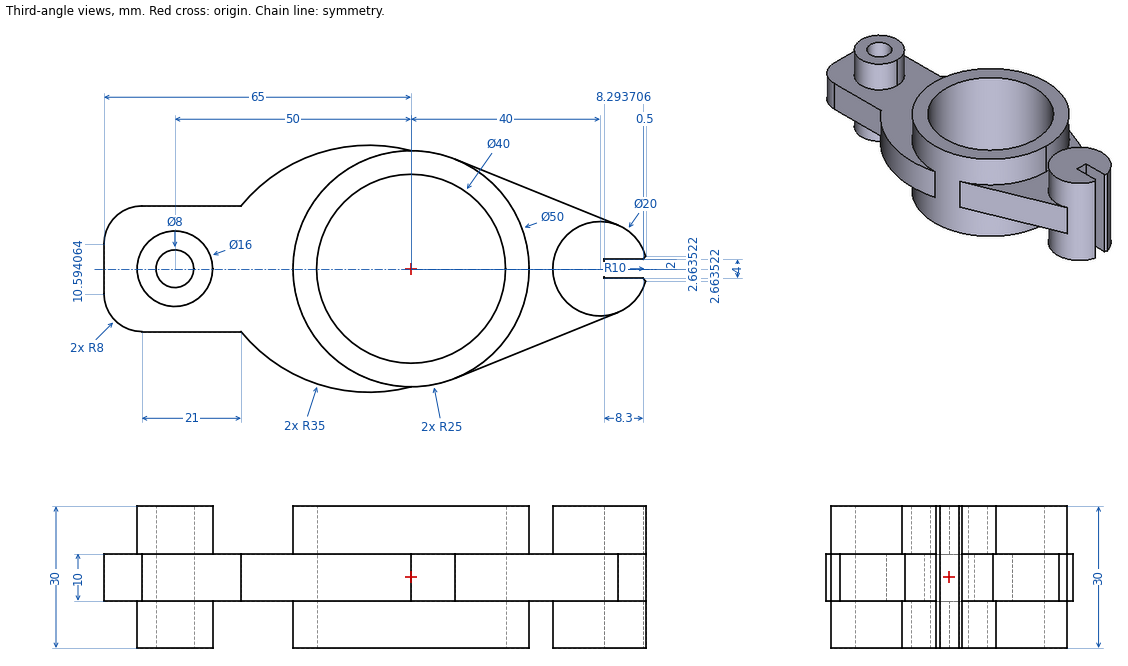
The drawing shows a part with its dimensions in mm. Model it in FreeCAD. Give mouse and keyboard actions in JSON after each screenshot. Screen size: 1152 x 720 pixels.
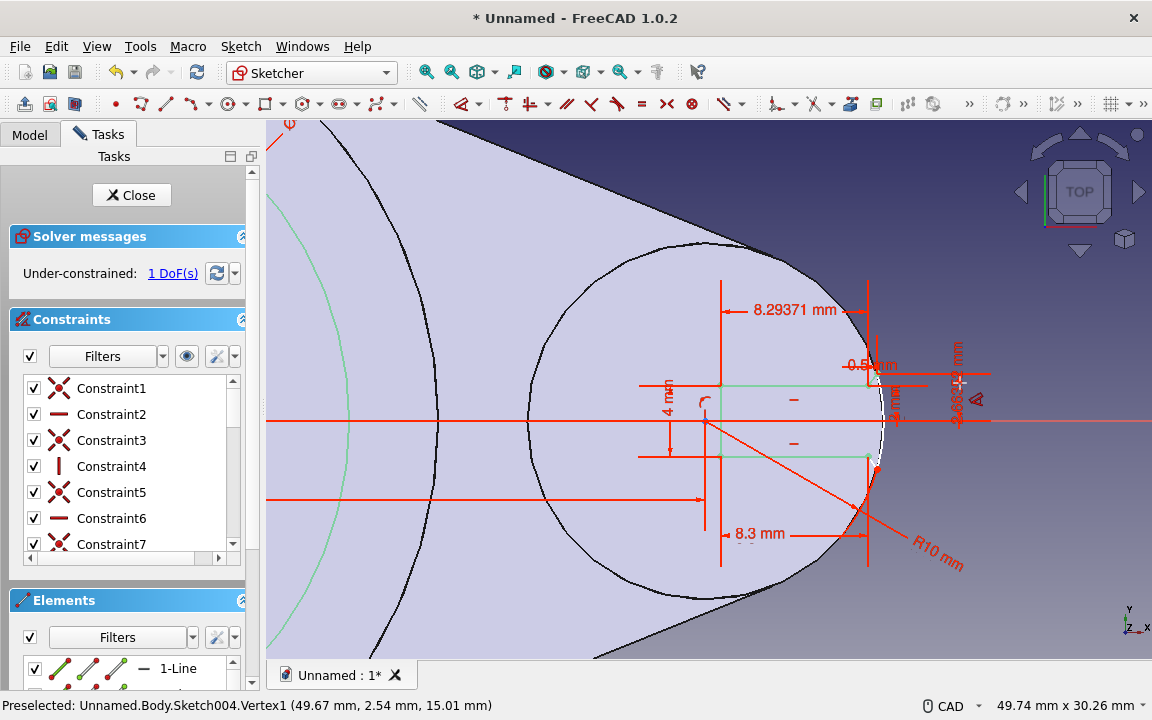
{"action": "left_click", "coordinate": [877, 469]}
{"action": "left_click", "coordinate": [911, 445]}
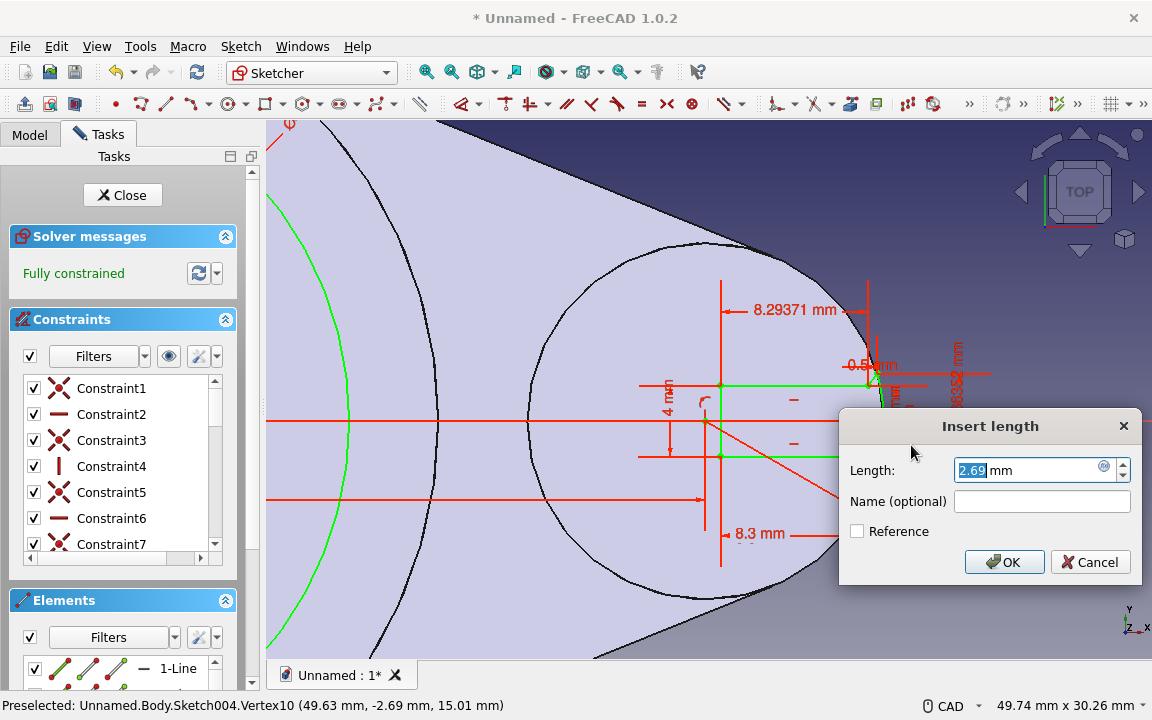
{"action": "type", "text": "2.663522"}
{"action": "key", "text": "Return"}
{"action": "key", "text": "Escape"}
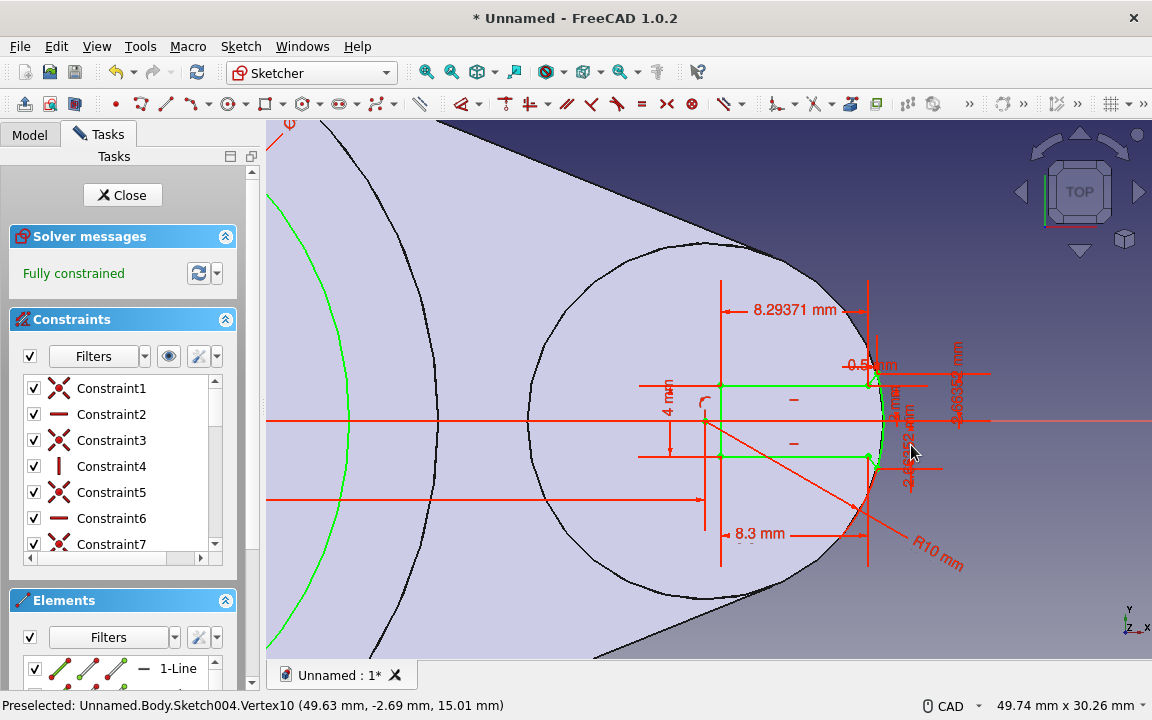
{"action": "left_click", "coordinate": [123, 195]}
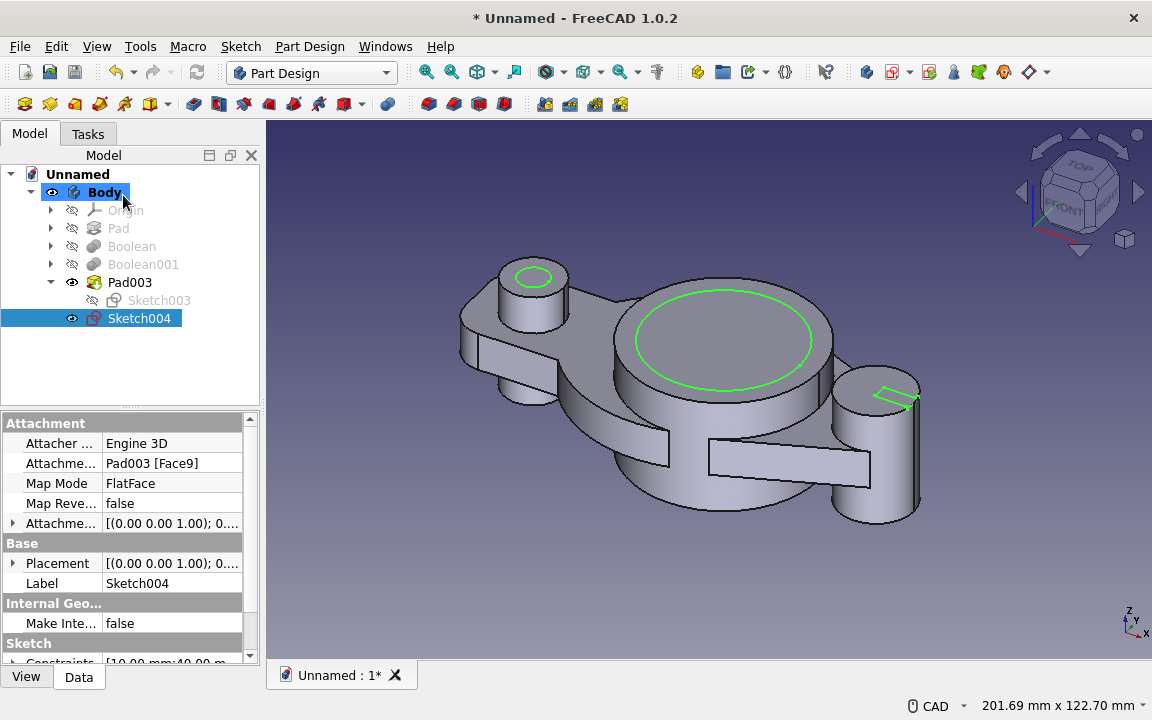
{"action": "left_click", "coordinate": [194, 104]}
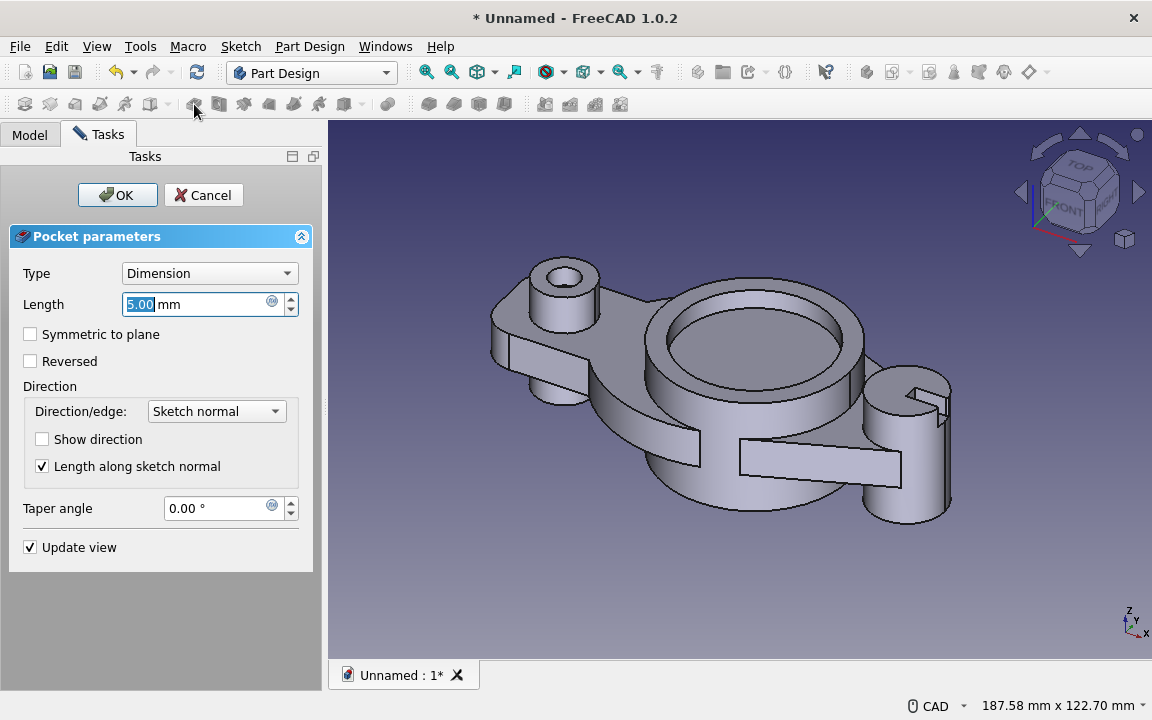
{"action": "left_click", "coordinate": [210, 274]}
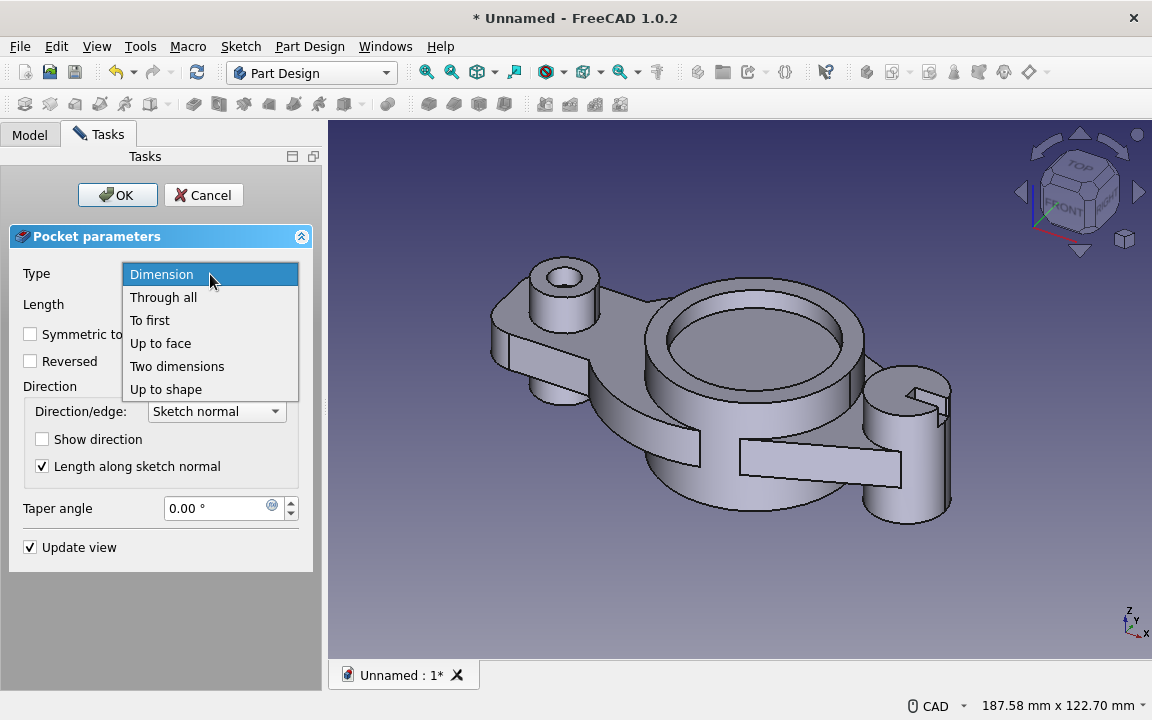
{"action": "left_click", "coordinate": [208, 298]}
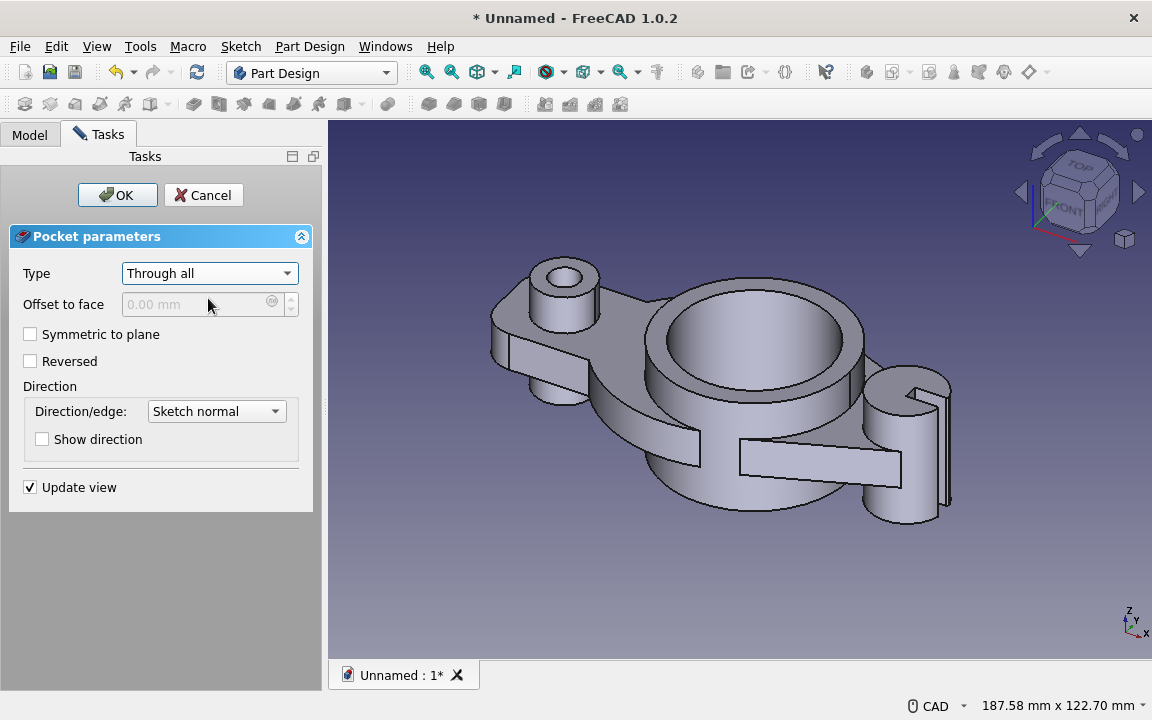
{"action": "left_click", "coordinate": [118, 195]}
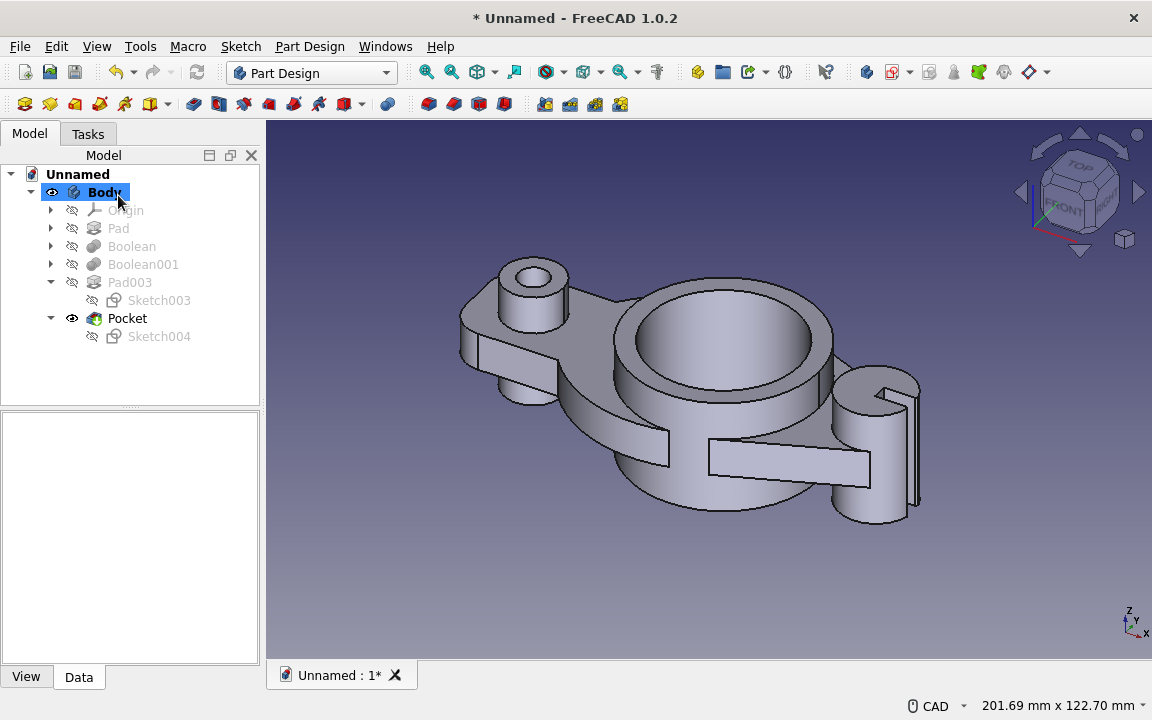
{"action": "key", "text": "0"}